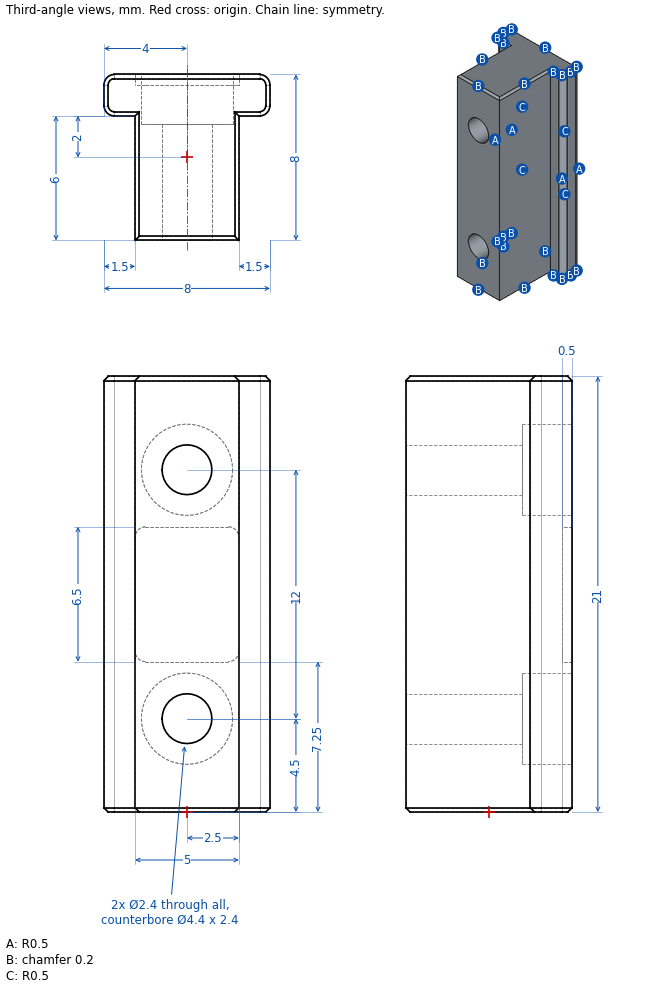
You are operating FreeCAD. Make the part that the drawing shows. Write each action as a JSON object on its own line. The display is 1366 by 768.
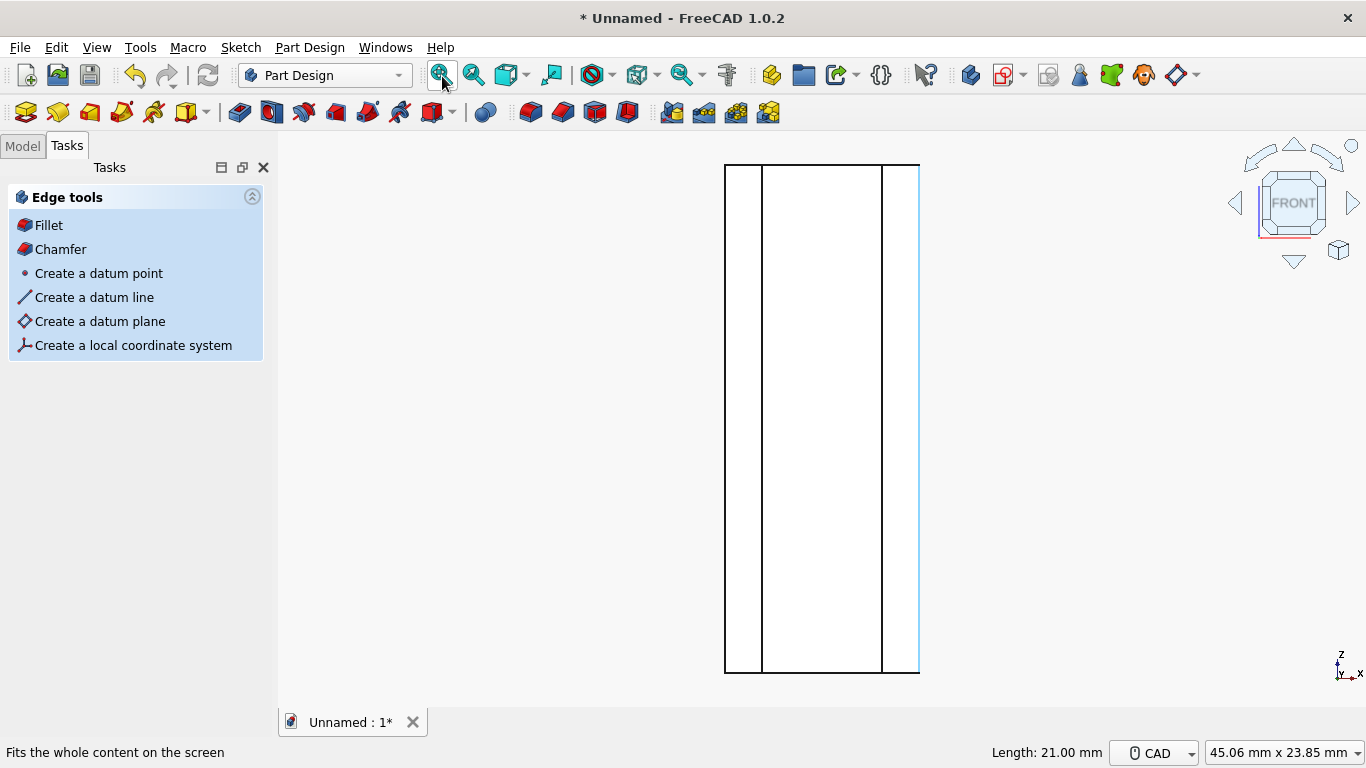
{"action": "left_click", "coordinate": [725, 418], "text": "ctrl"}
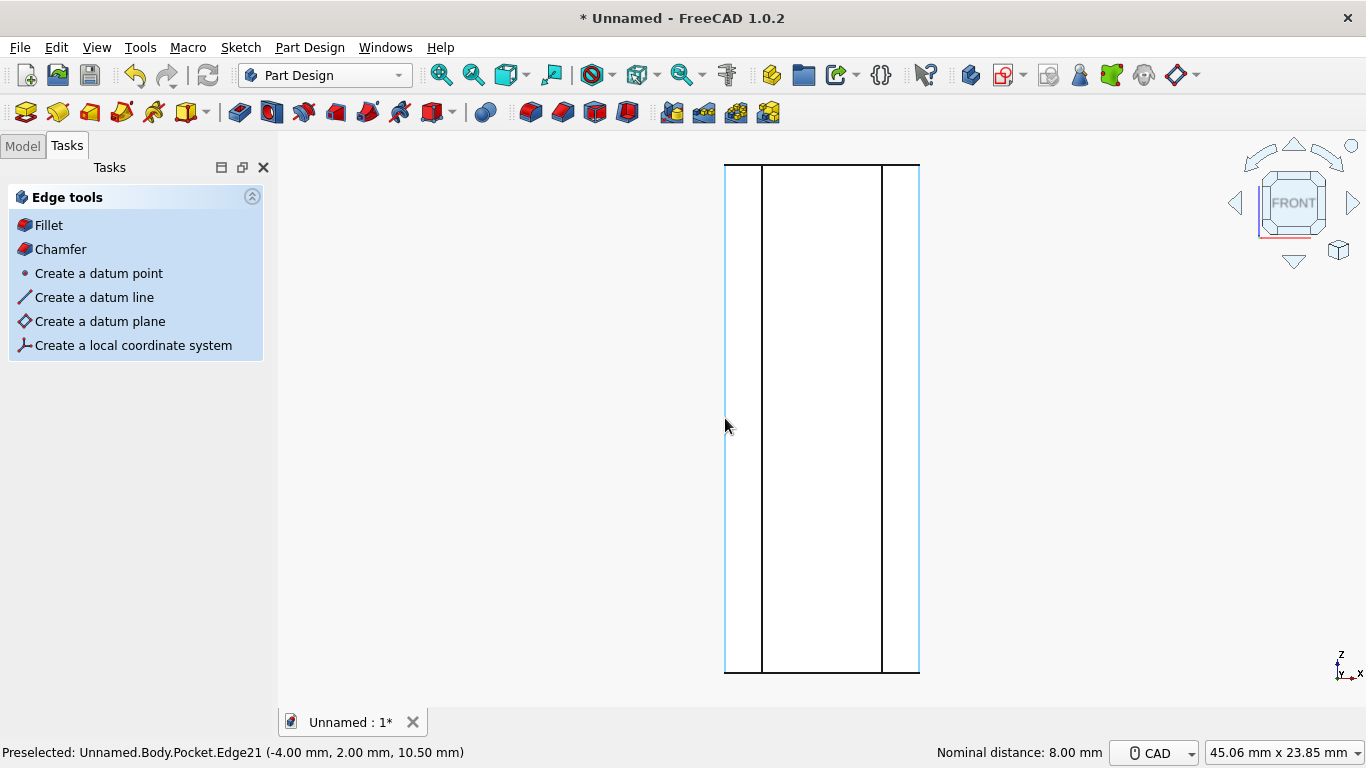
{"action": "key", "text": "3"}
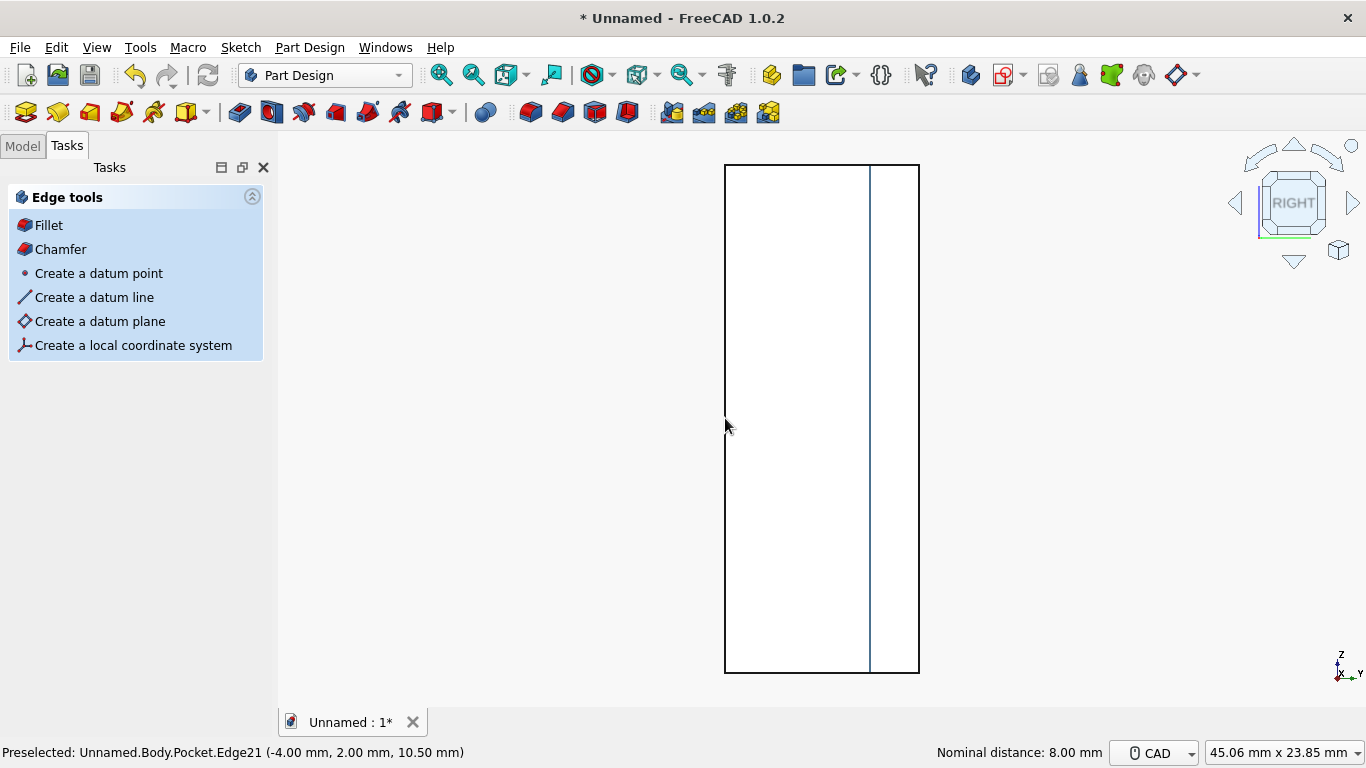
{"action": "left_click", "coordinate": [919, 418], "text": "ctrl"}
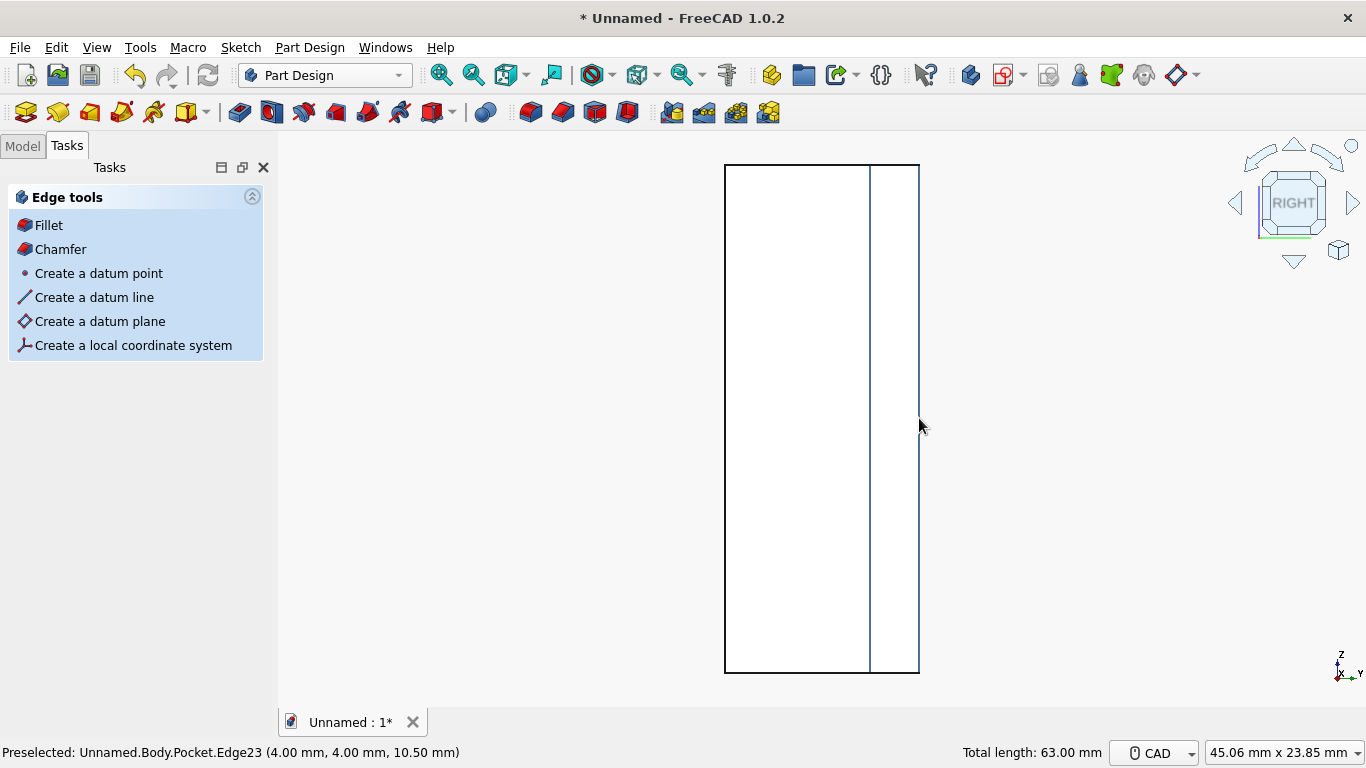
{"action": "key", "text": "5"}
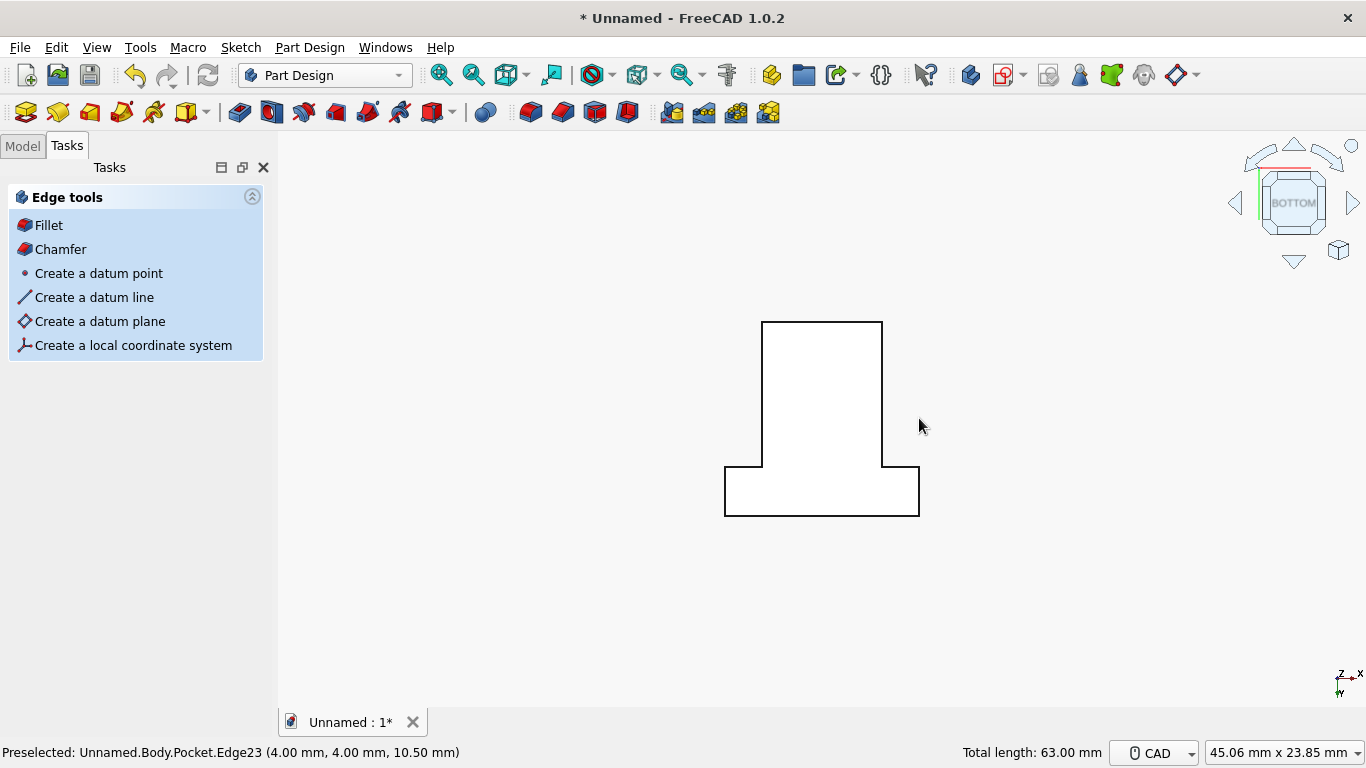
{"action": "left_click", "coordinate": [442, 76]}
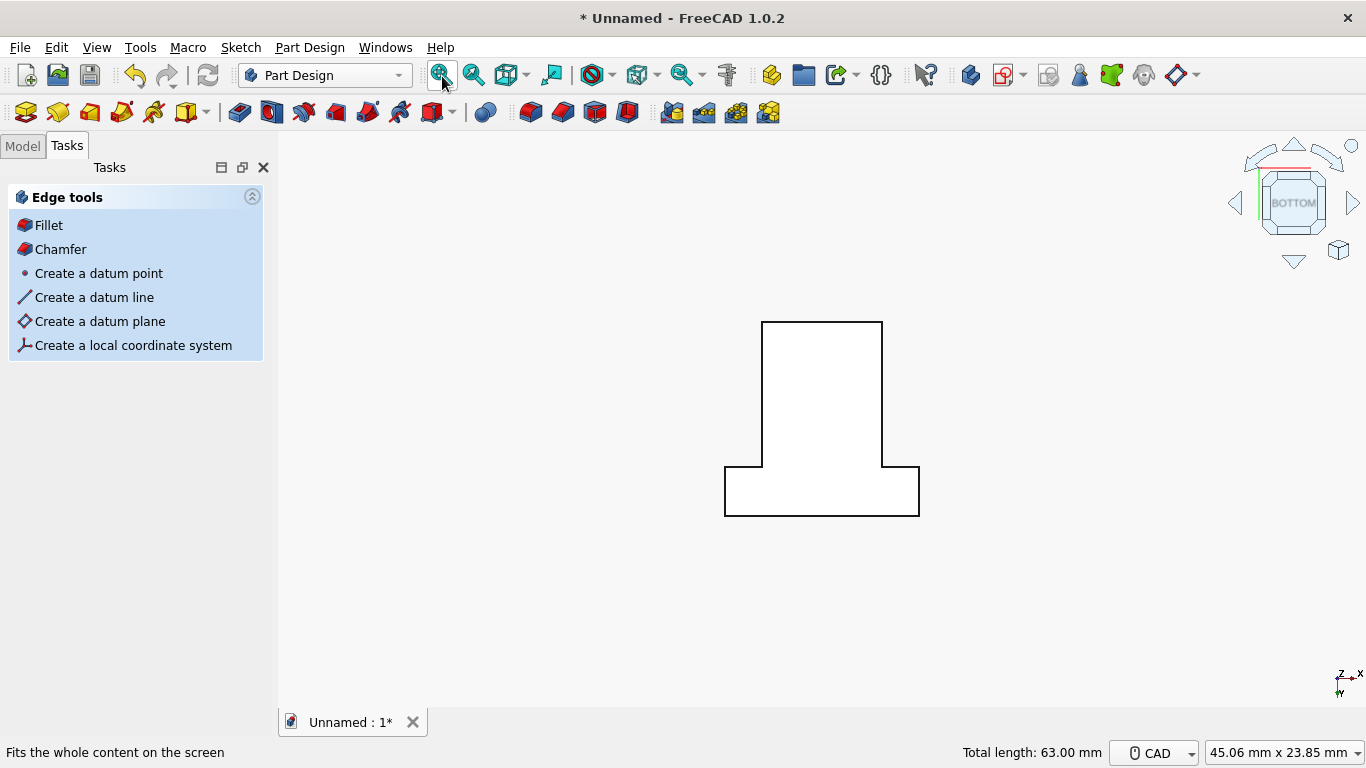
{"action": "key", "text": "4"}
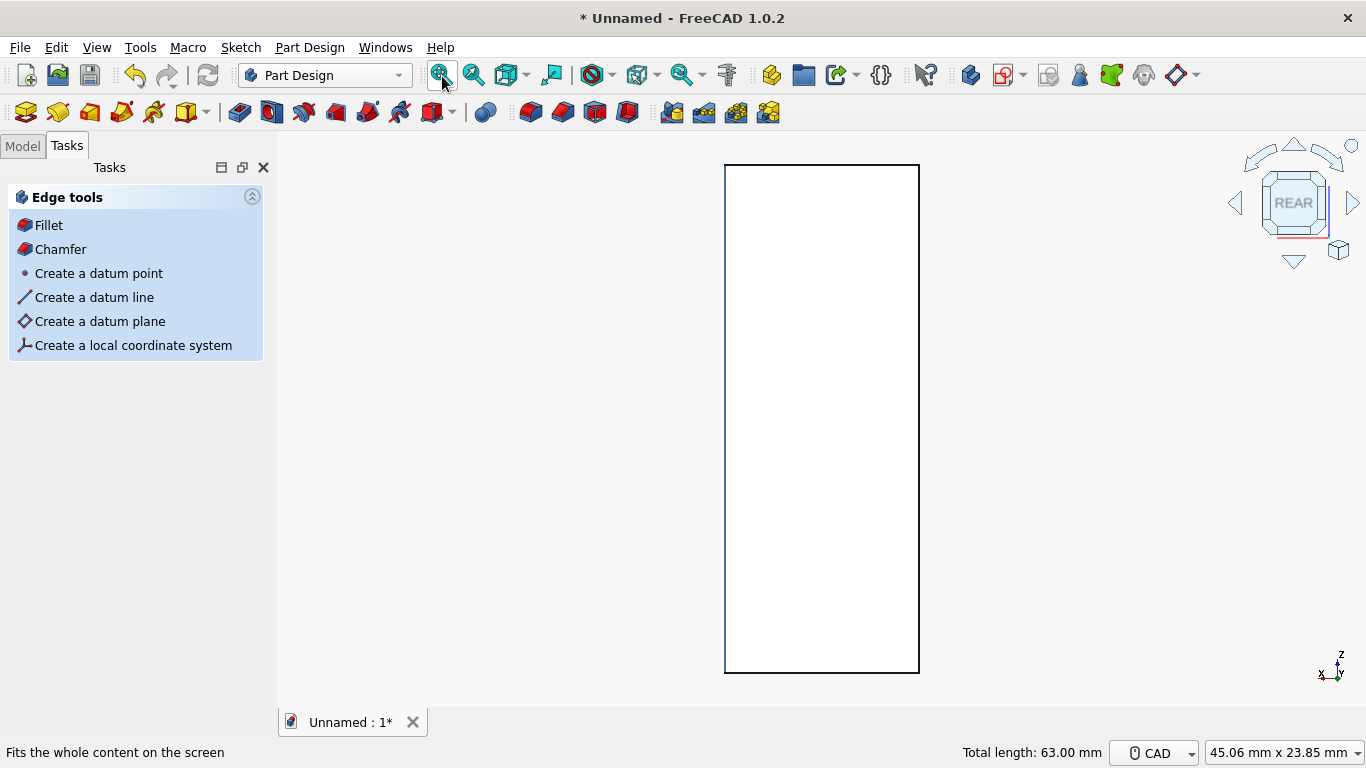
{"action": "left_click", "coordinate": [919, 418], "text": "ctrl"}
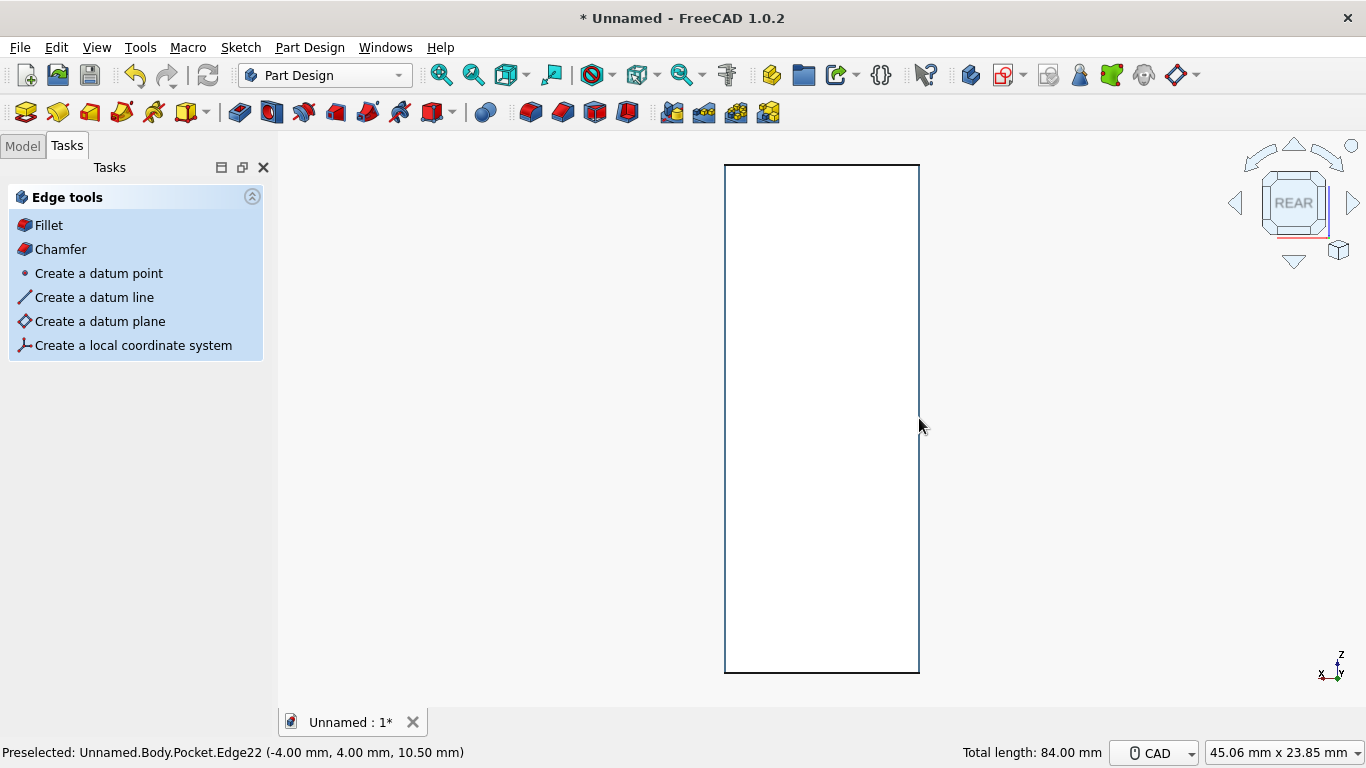
{"action": "left_click", "coordinate": [532, 112]}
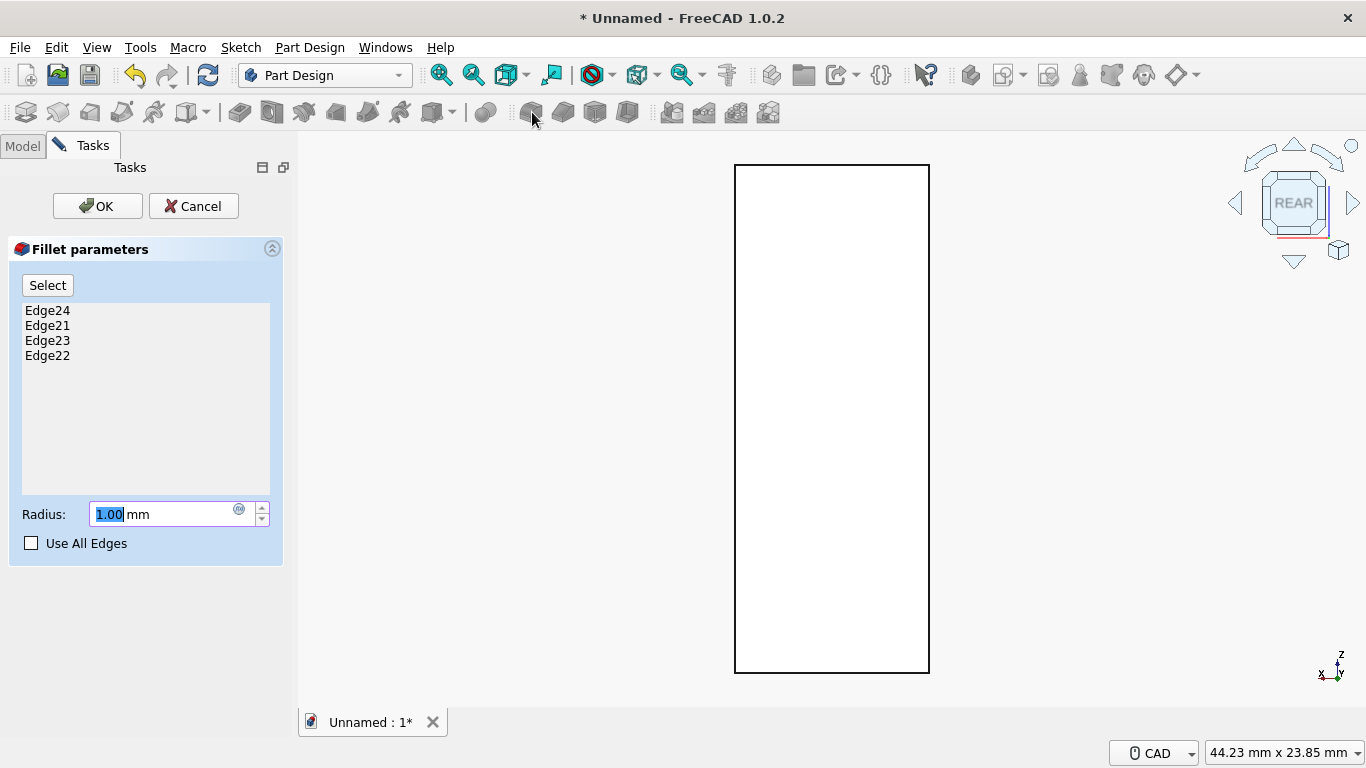
{"action": "type", "text": "0.5"}
{"action": "key", "text": "Tab"}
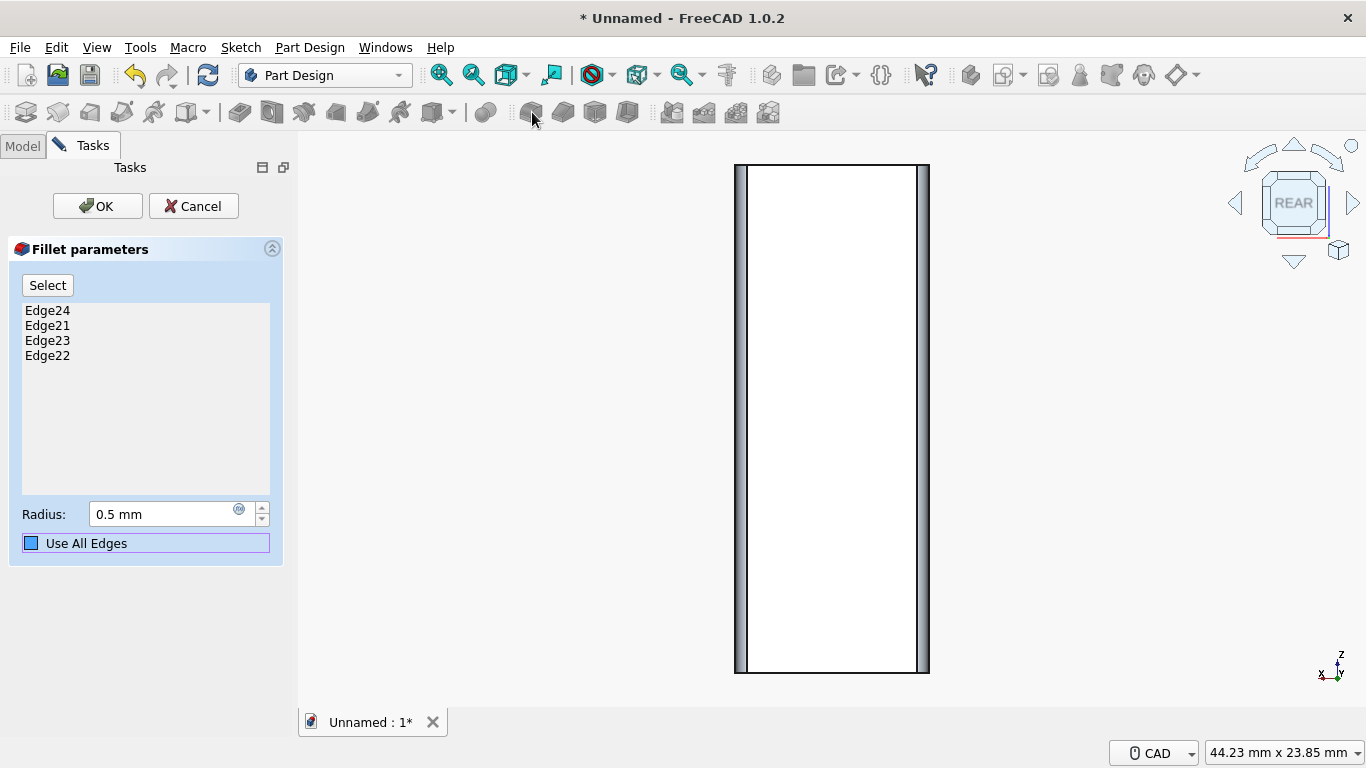
{"action": "left_click", "coordinate": [98, 206]}